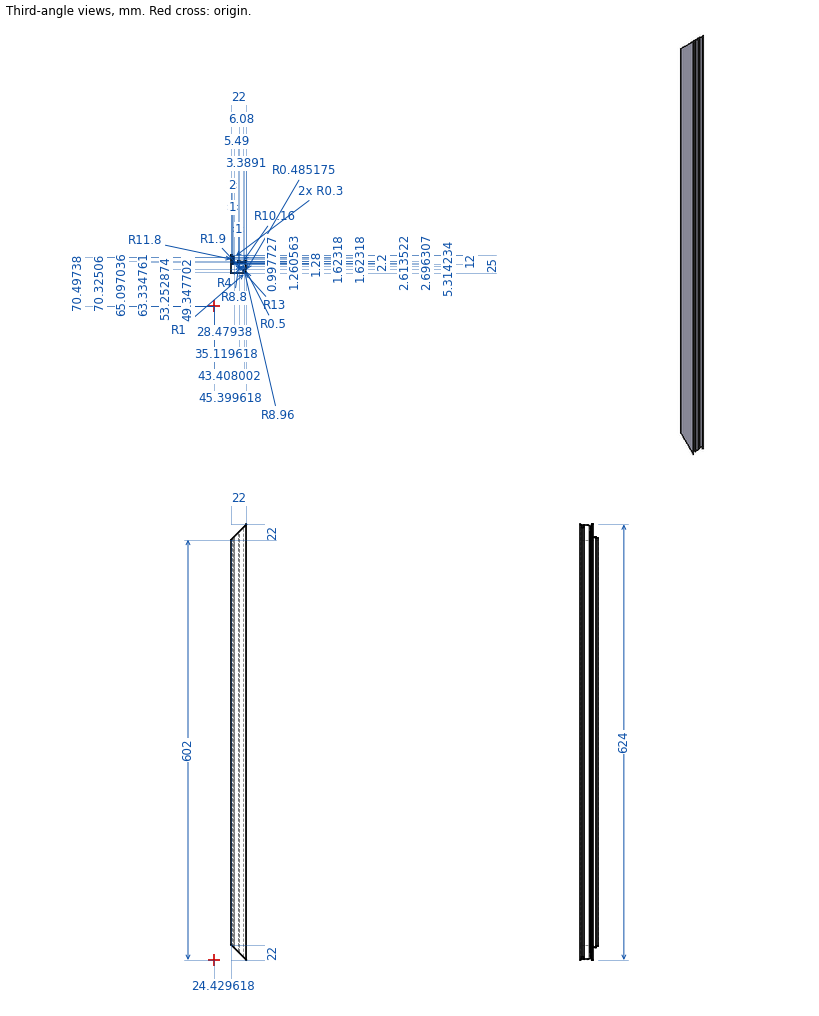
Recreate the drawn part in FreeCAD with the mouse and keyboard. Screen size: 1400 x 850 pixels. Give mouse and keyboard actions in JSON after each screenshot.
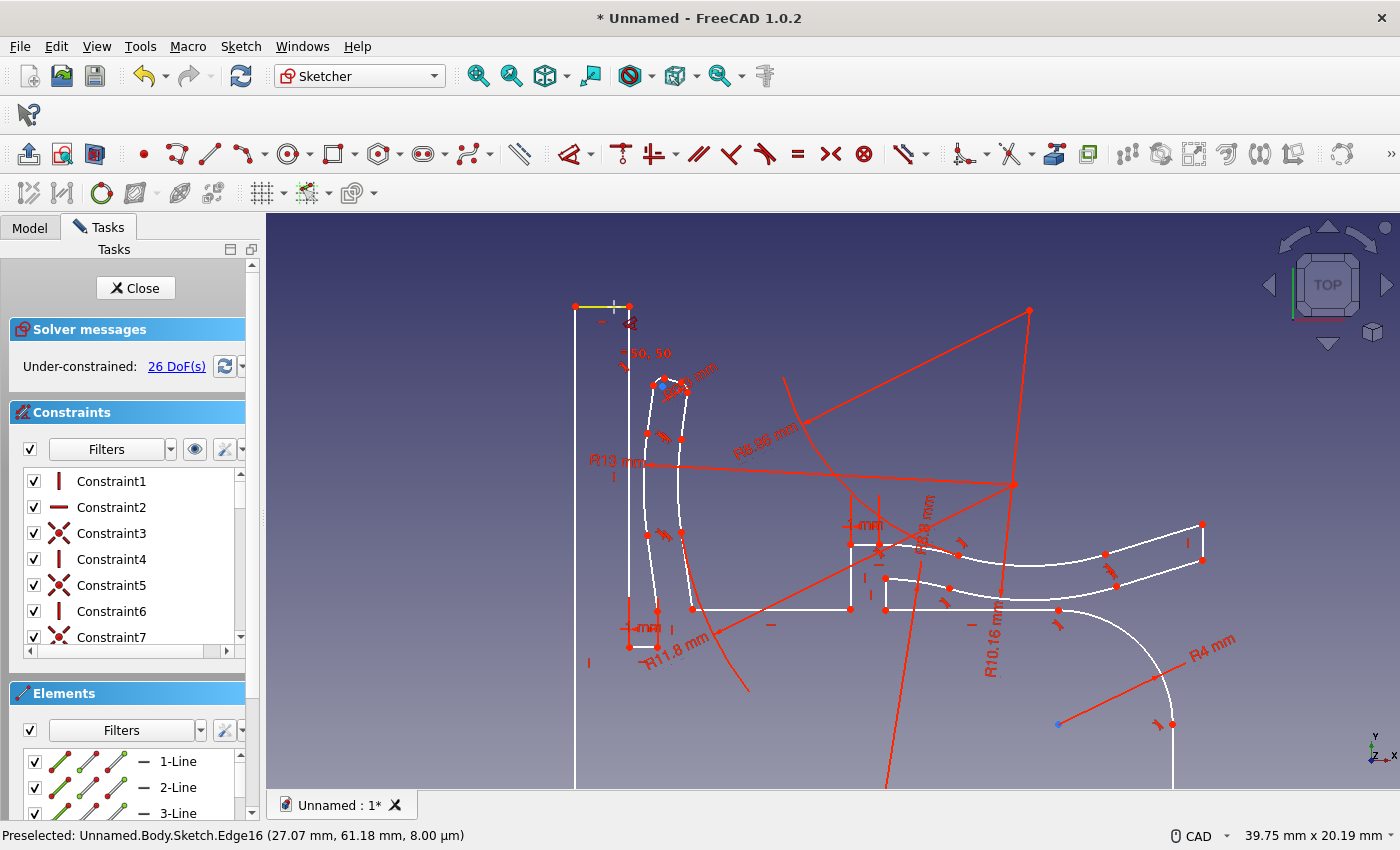
{"action": "left_click", "coordinate": [613, 307]}
{"action": "left_click", "coordinate": [602, 273]}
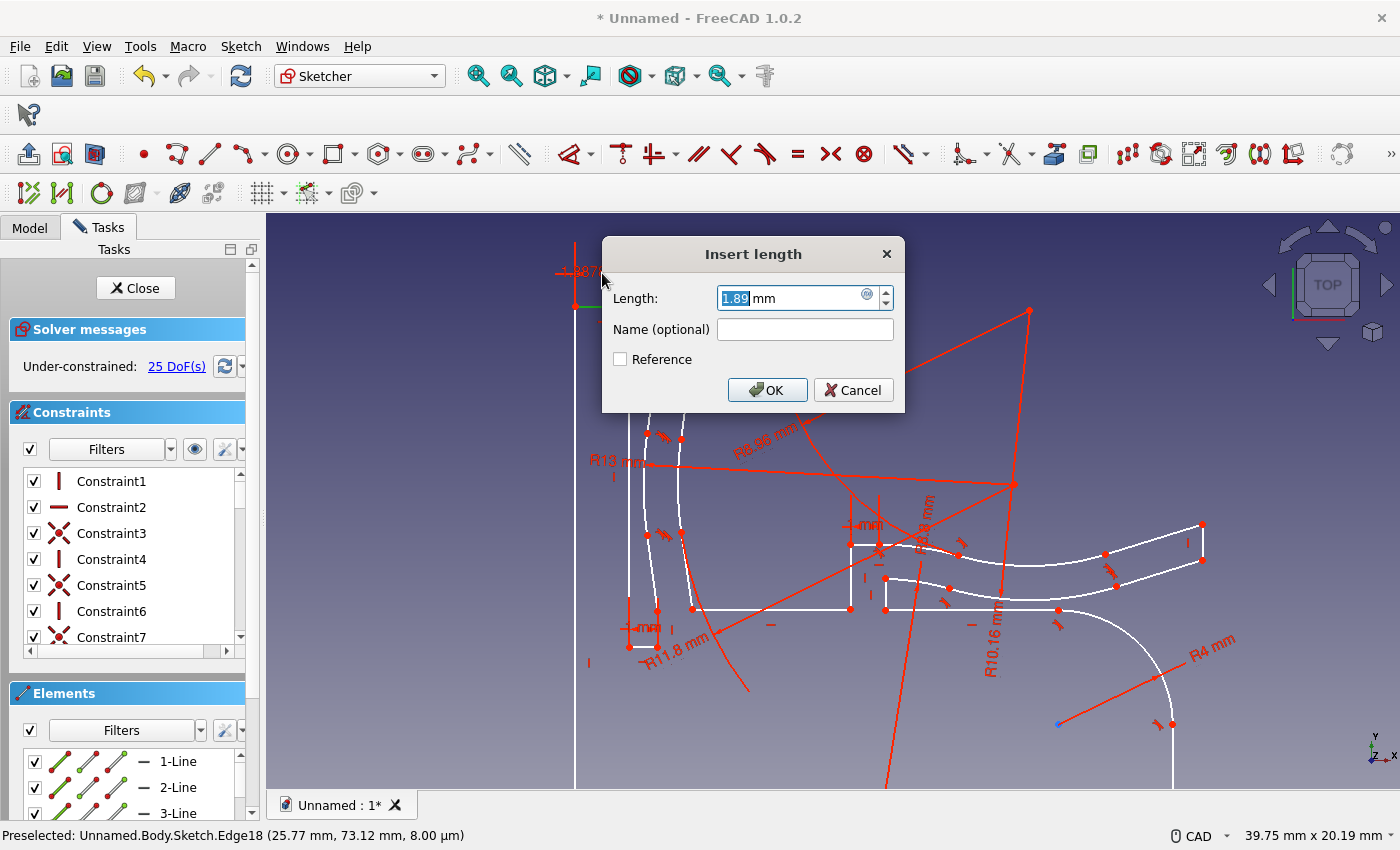
{"action": "type", "text": "2"}
{"action": "key", "text": "Return"}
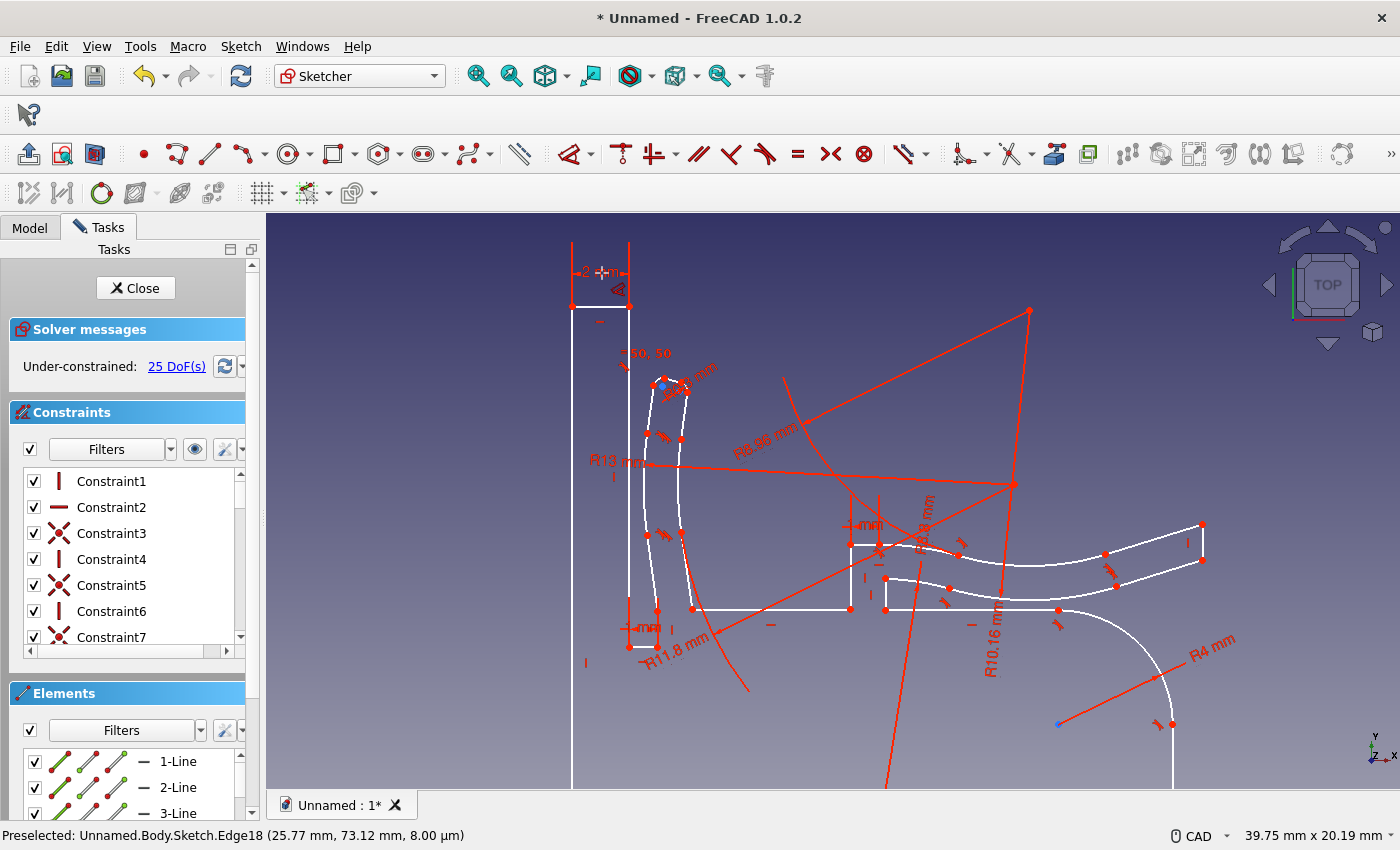
{"action": "left_click", "coordinate": [629, 545]}
{"action": "left_click", "coordinate": [595, 399]}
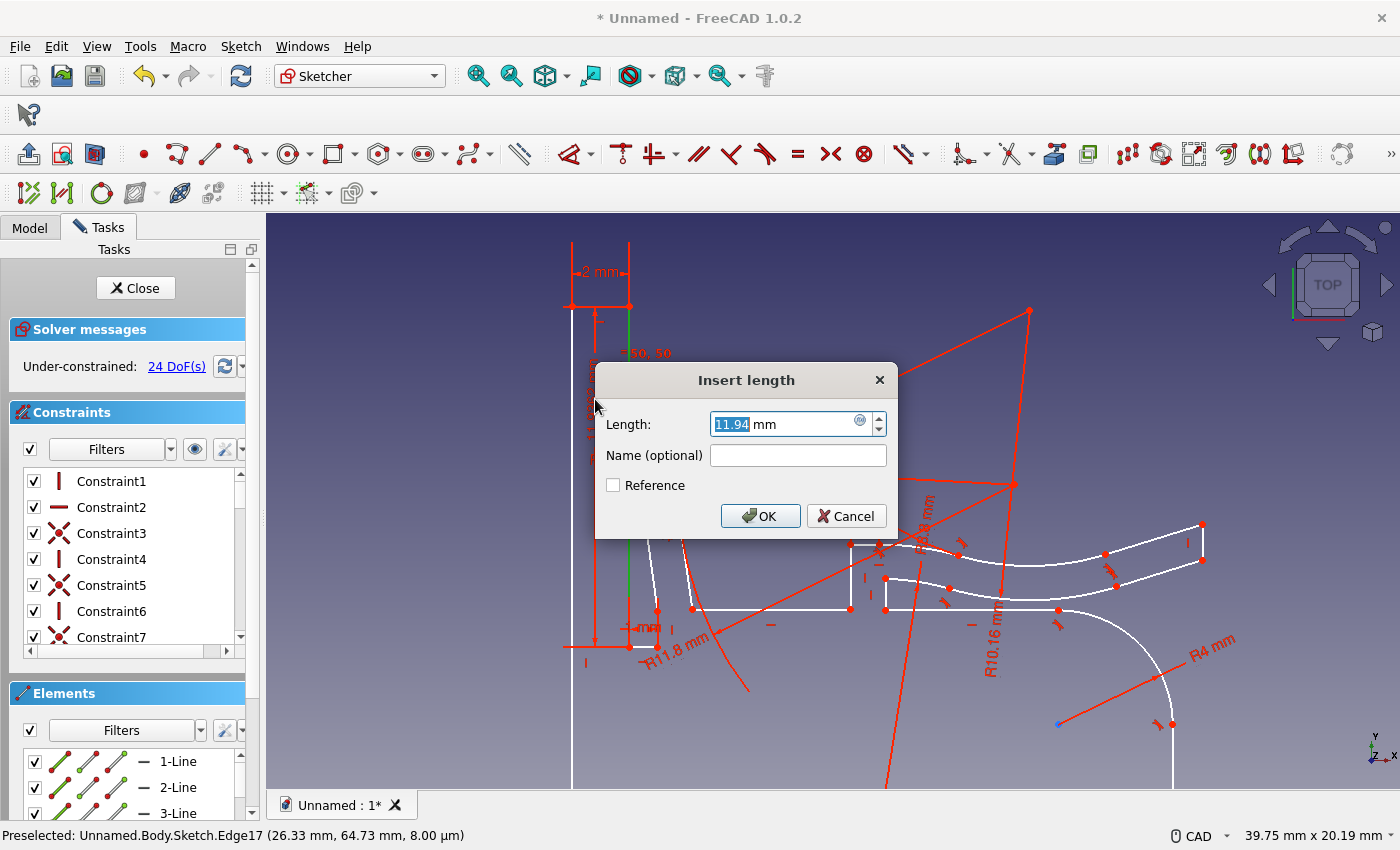
{"action": "type", "text": "12"}
{"action": "key", "text": "Return"}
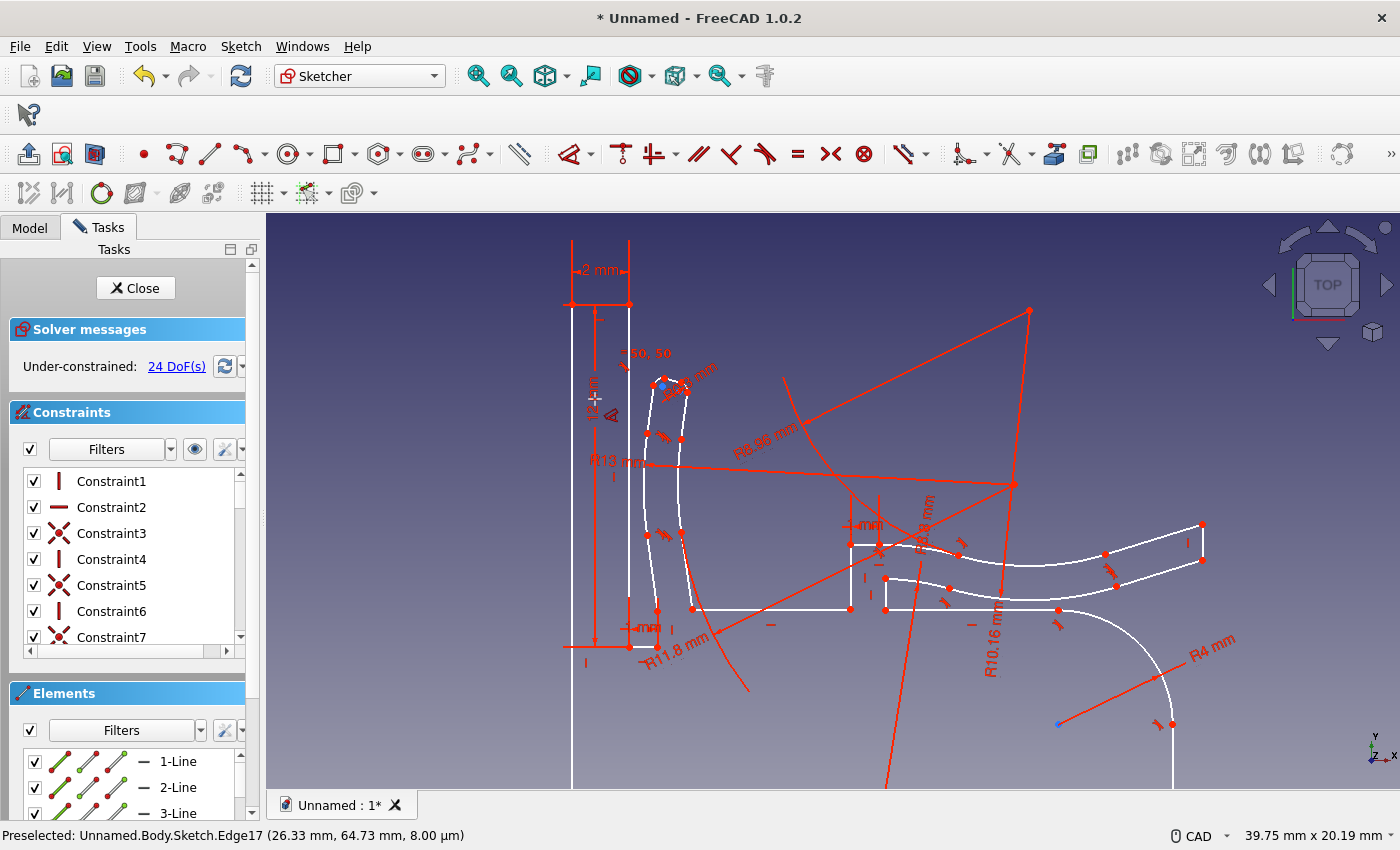
{"action": "left_click", "coordinate": [572, 519]}
{"action": "left_click", "coordinate": [538, 533]}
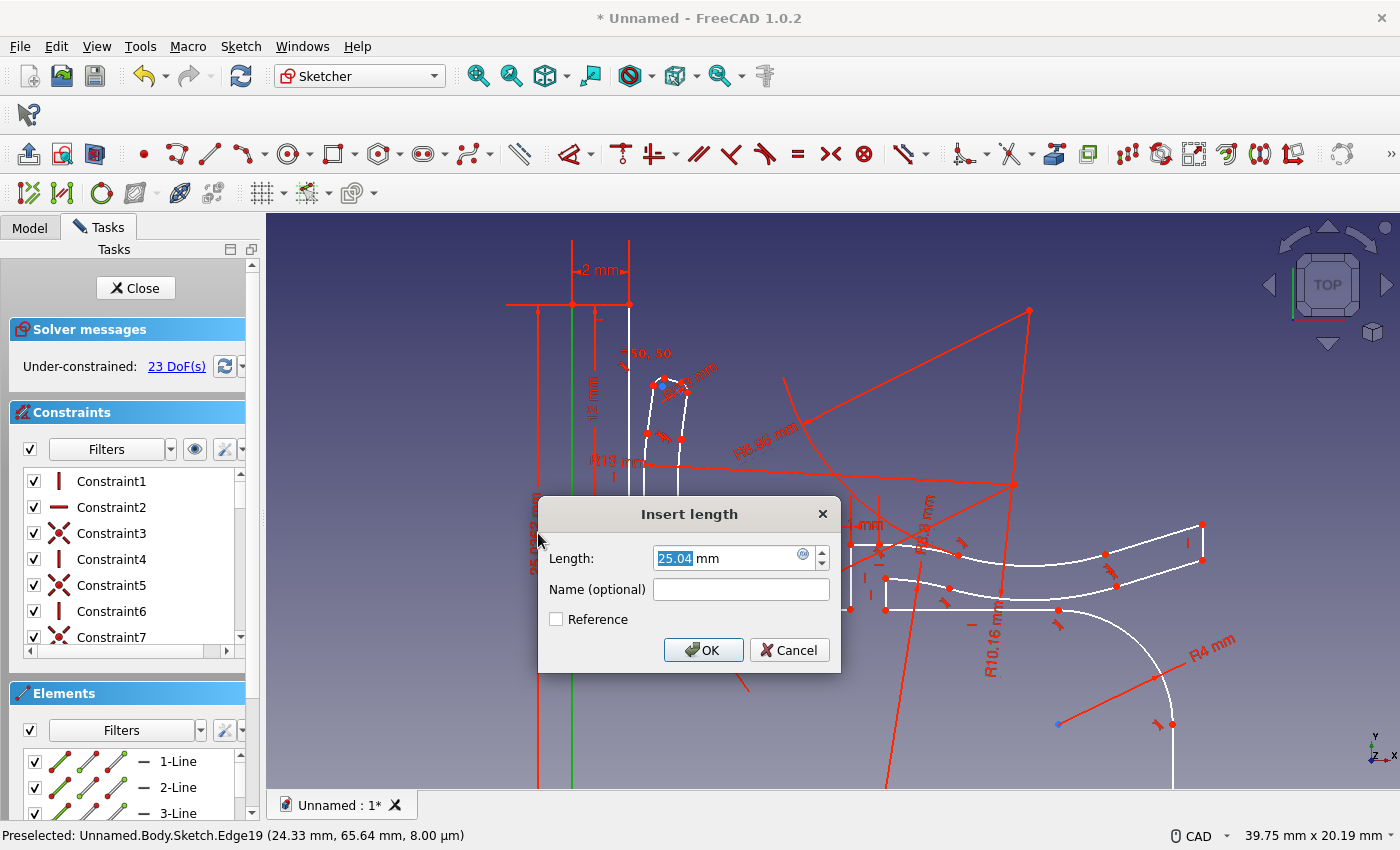
{"action": "type", "text": "25"}
{"action": "key", "text": "Return"}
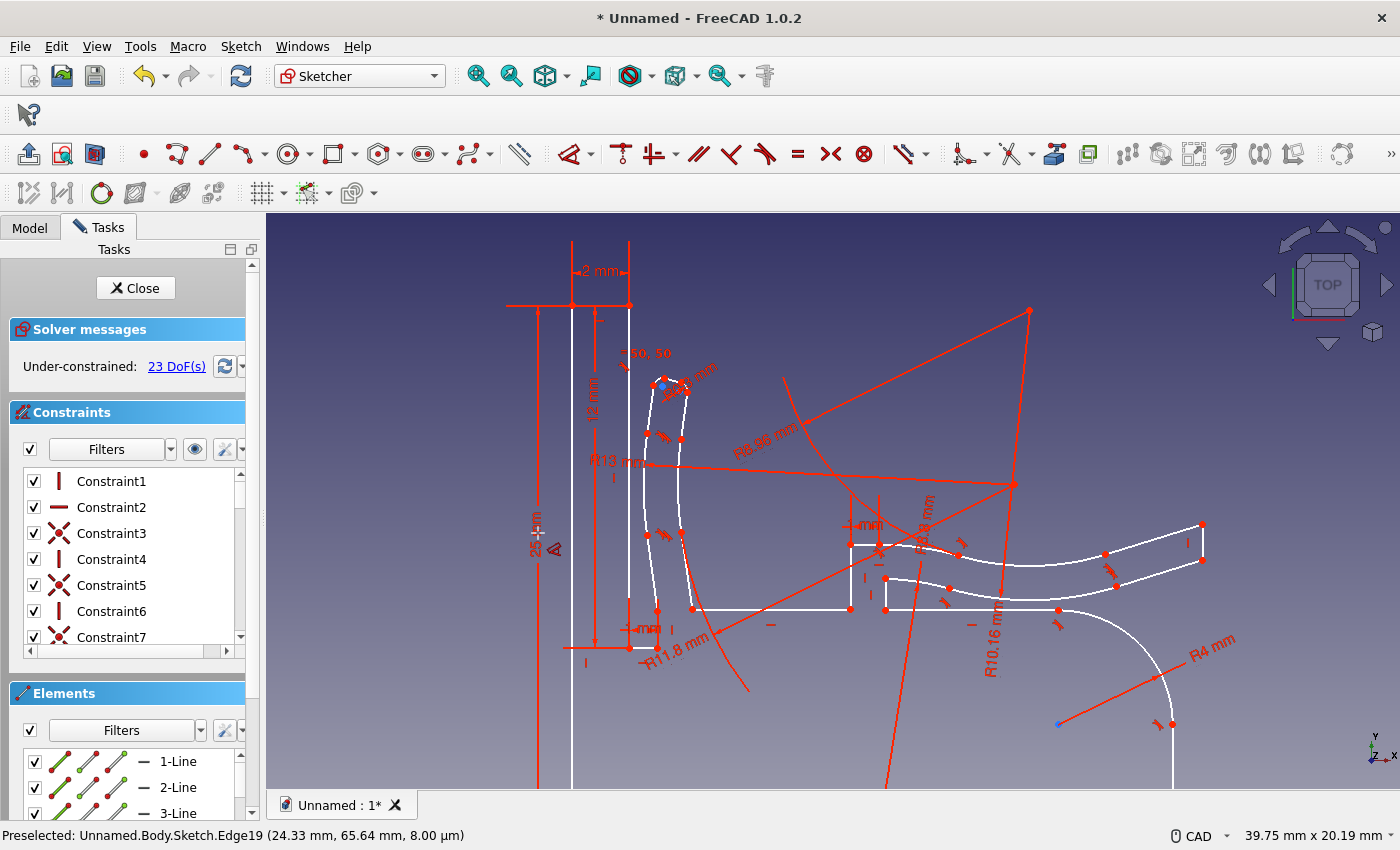
{"action": "scroll", "coordinate": [613, 307], "scroll_direction": "down", "scroll_amount": 3}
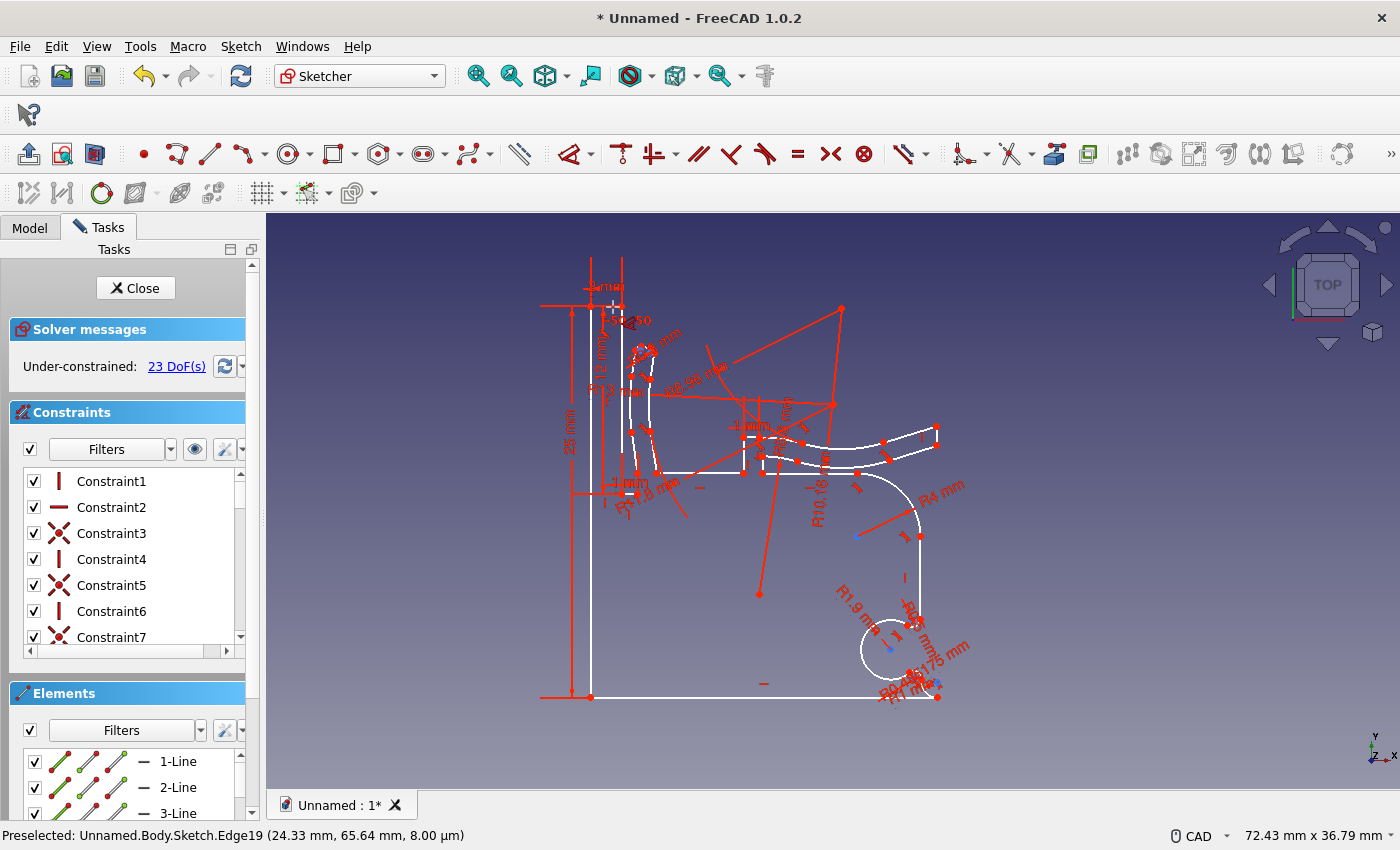
{"action": "left_click", "coordinate": [695, 698]}
{"action": "left_click", "coordinate": [764, 732]}